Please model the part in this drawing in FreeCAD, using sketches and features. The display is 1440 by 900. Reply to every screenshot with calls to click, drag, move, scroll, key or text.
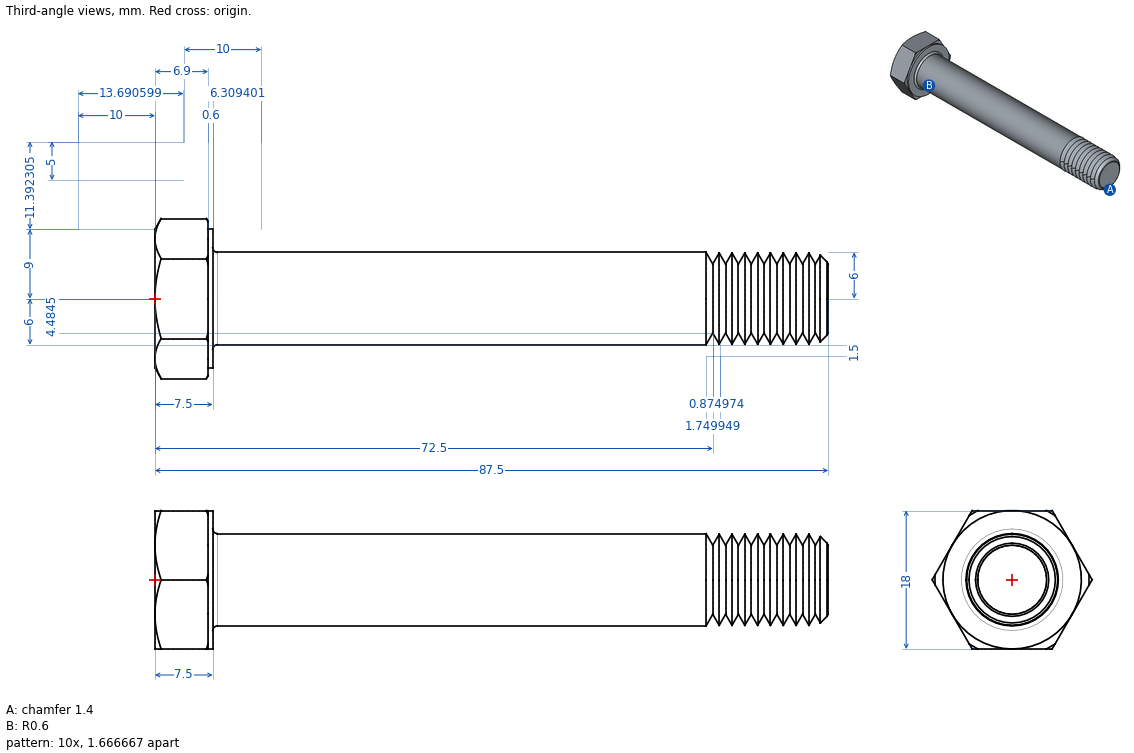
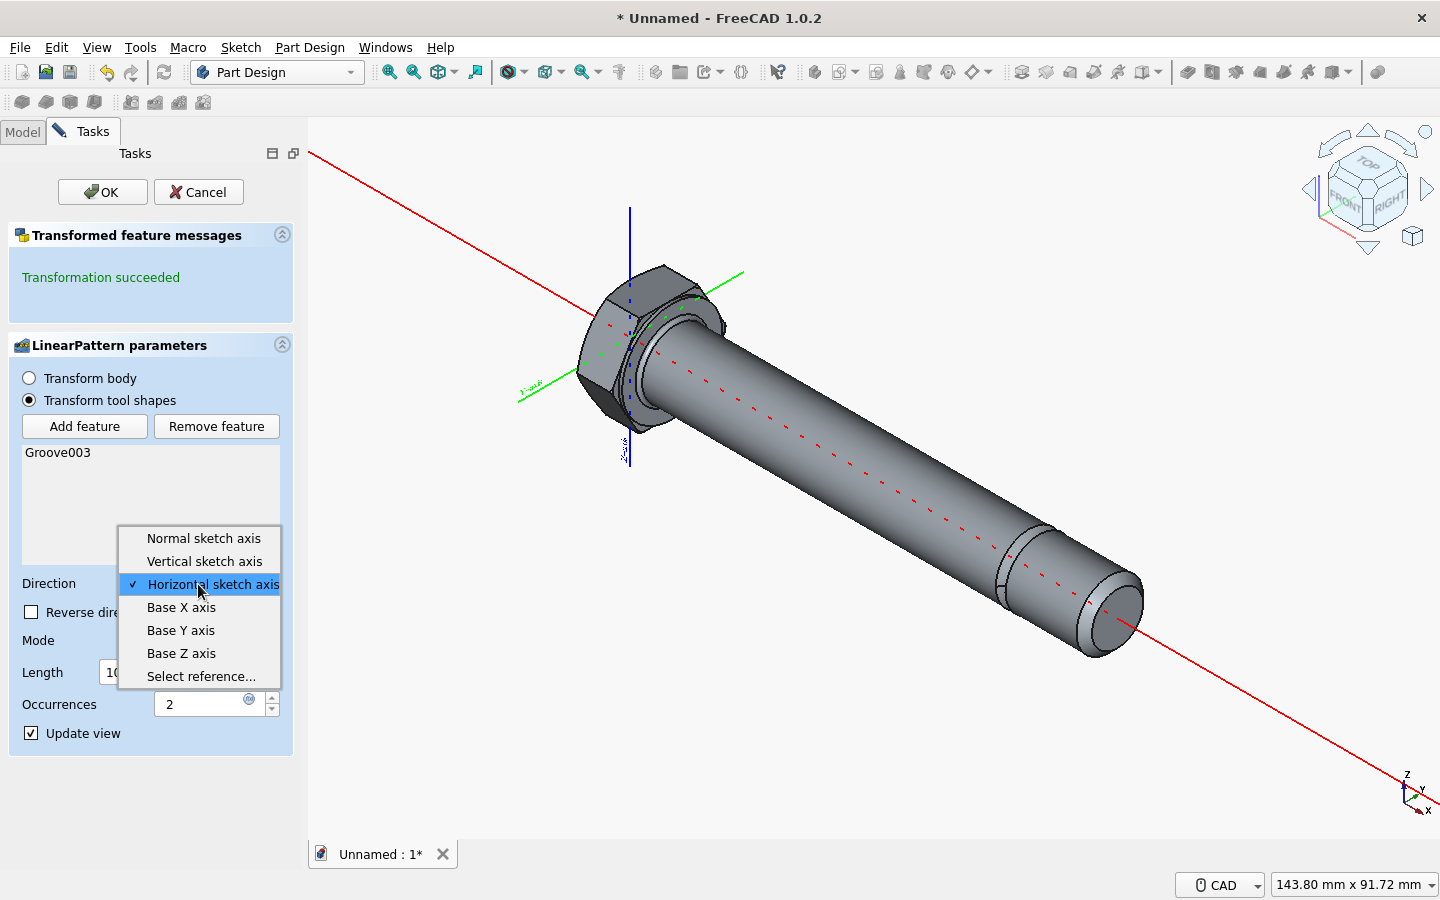
click(198, 608)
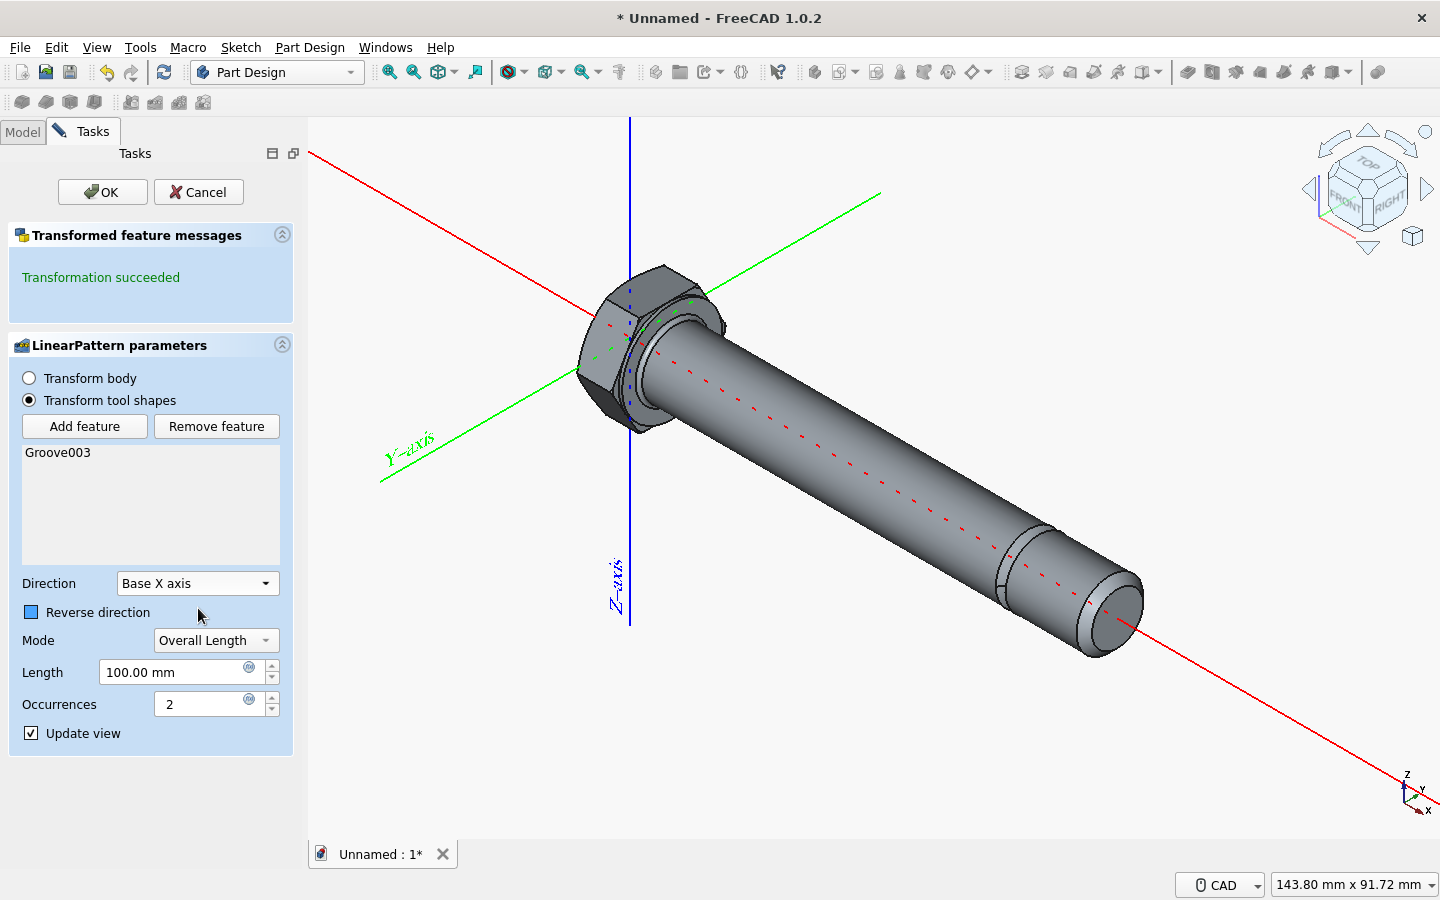
click(217, 640)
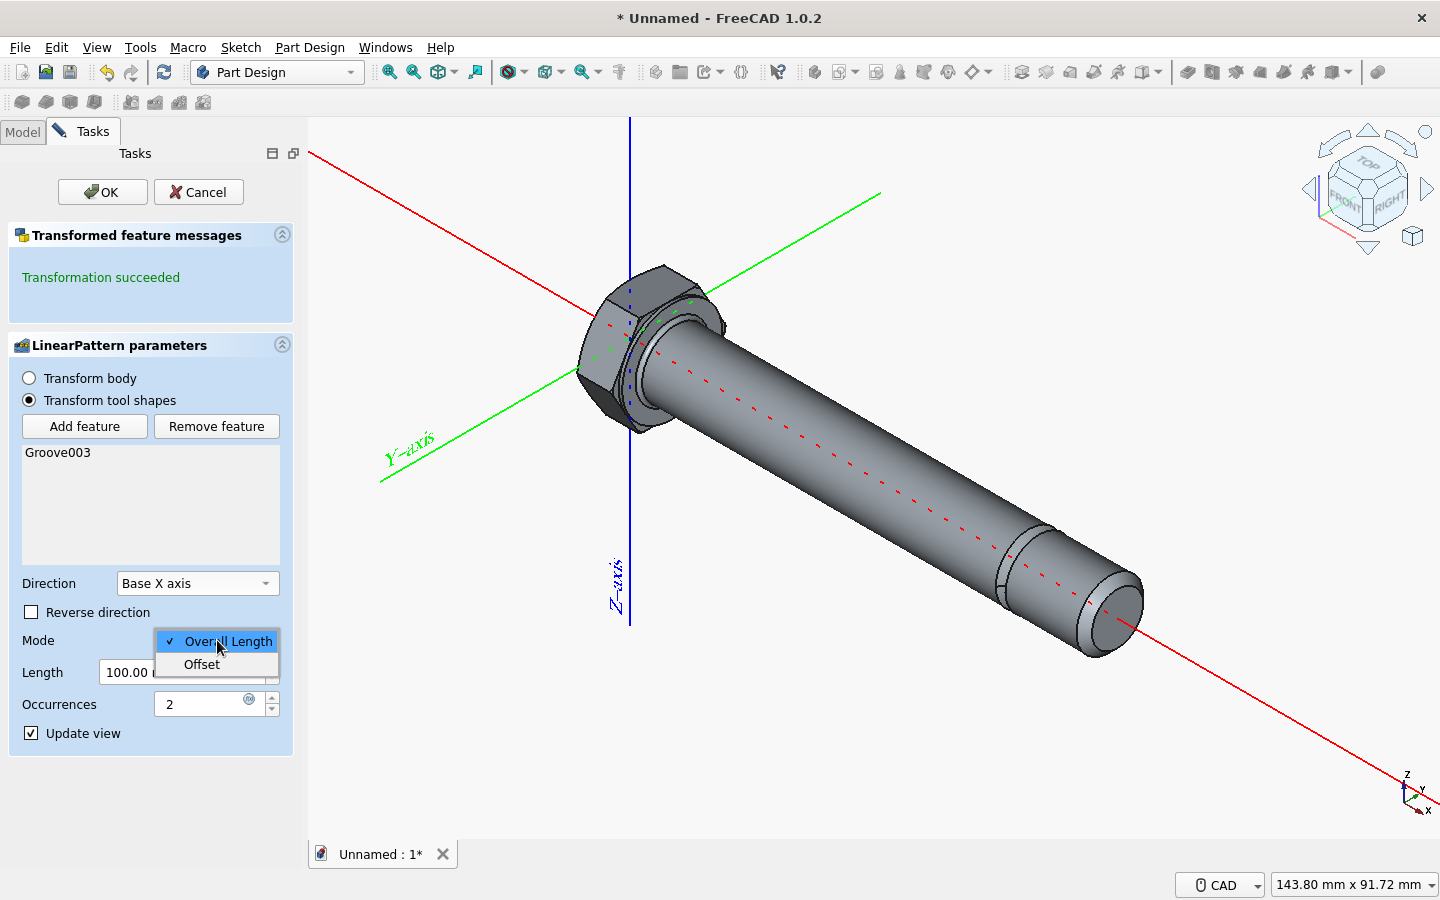
click(216, 664)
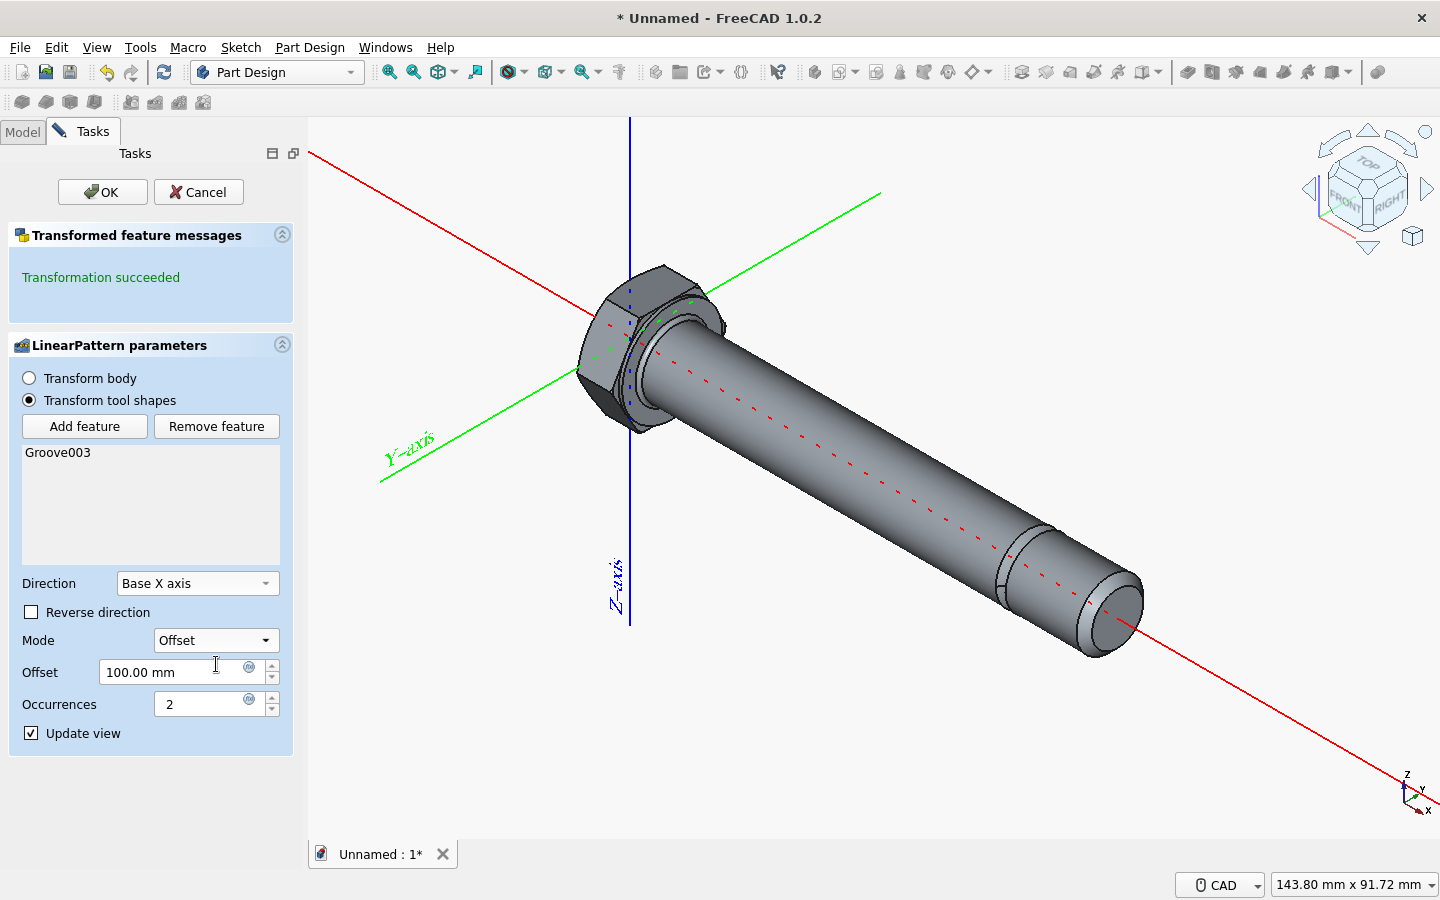
triple_click(182, 672)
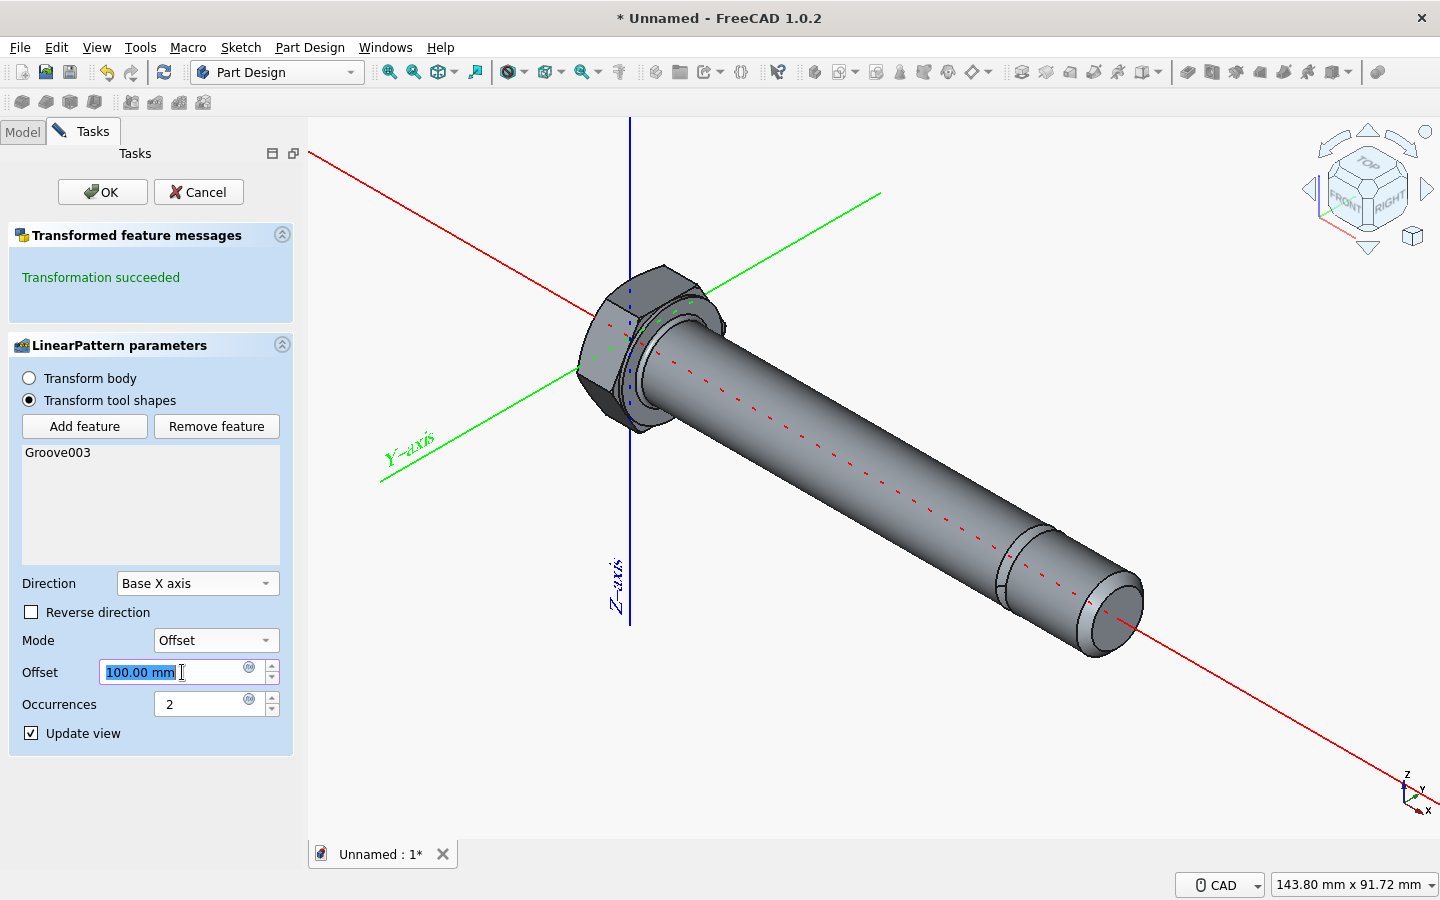
text(1.666667)
key(Tab)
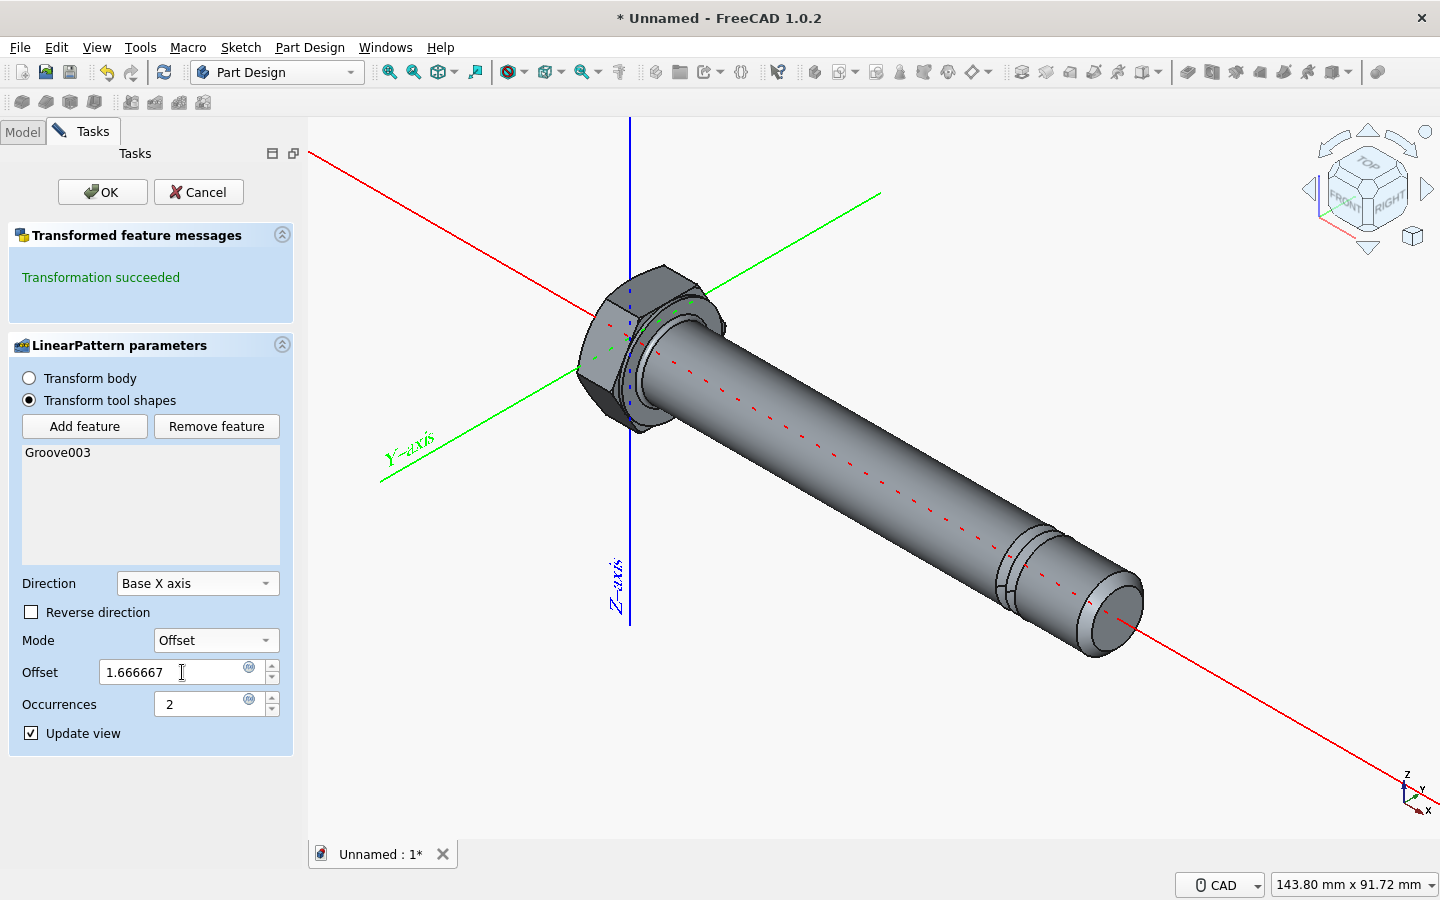
triple_click(209, 704)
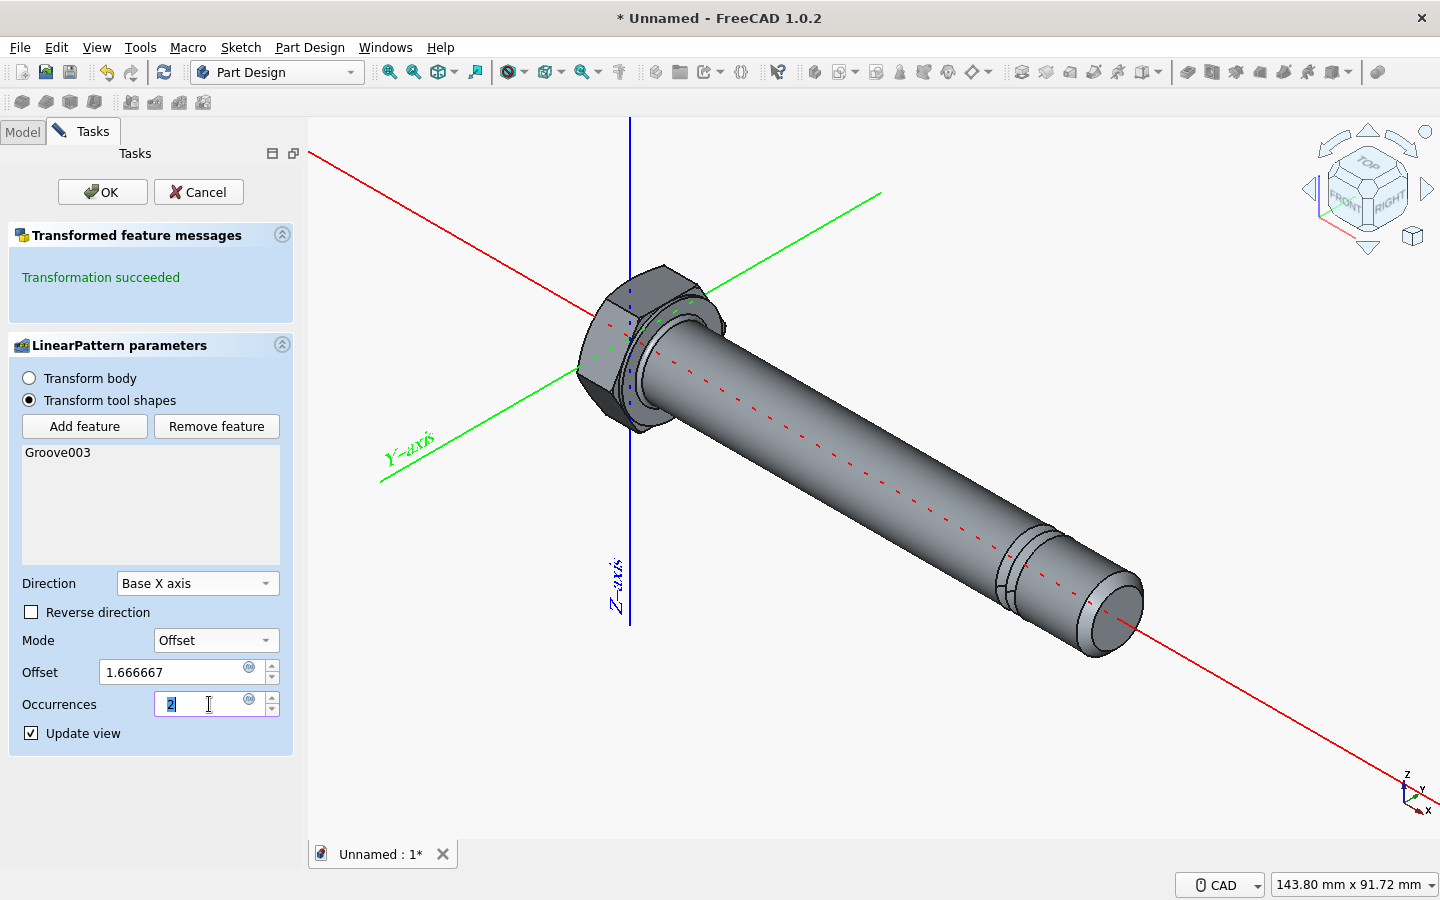
text(10)
key(Tab)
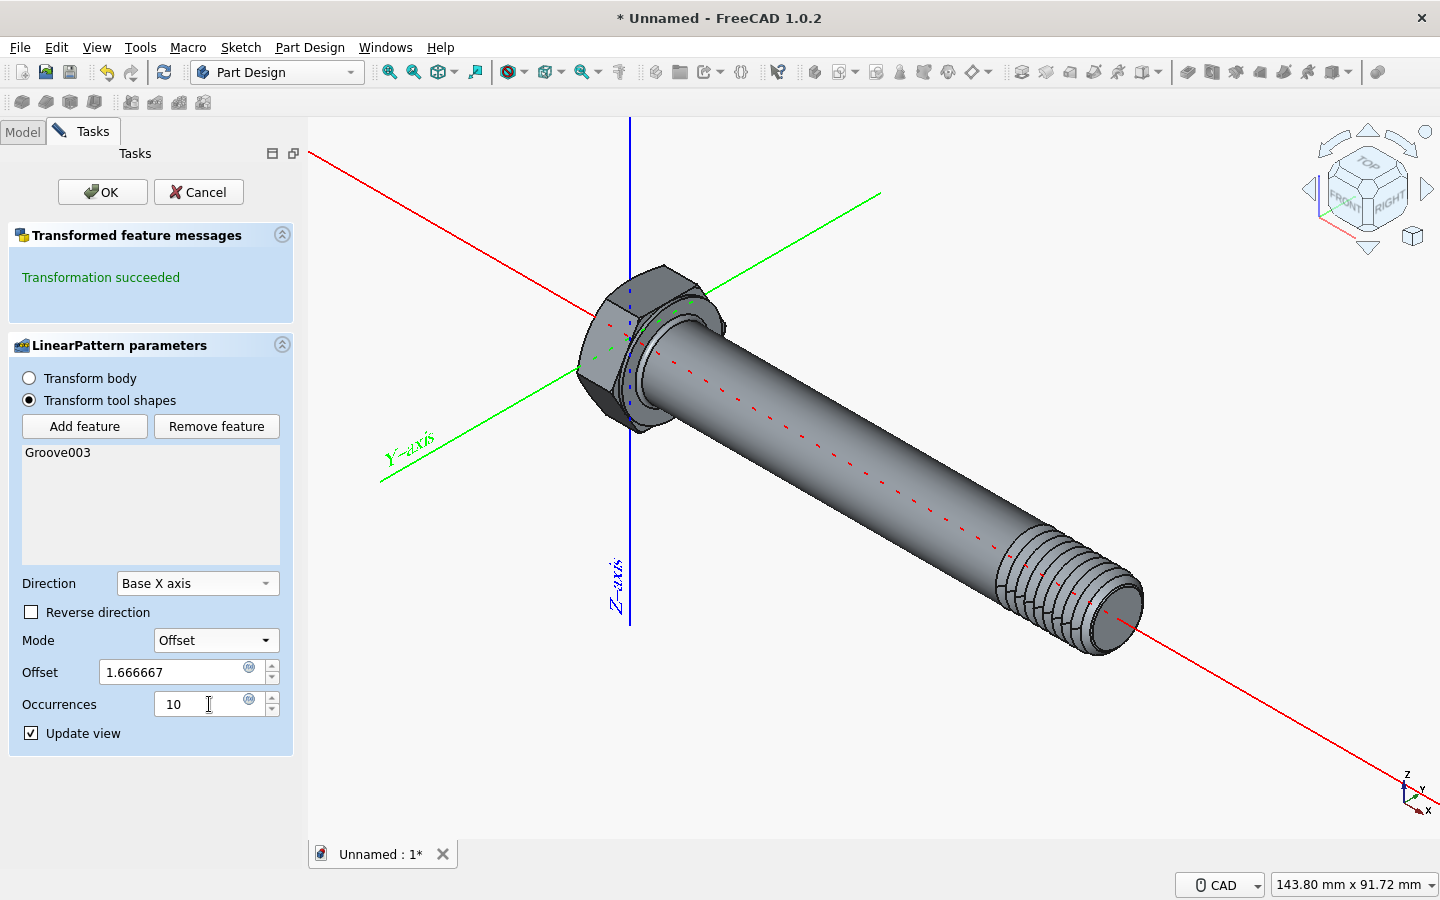
click(103, 192)